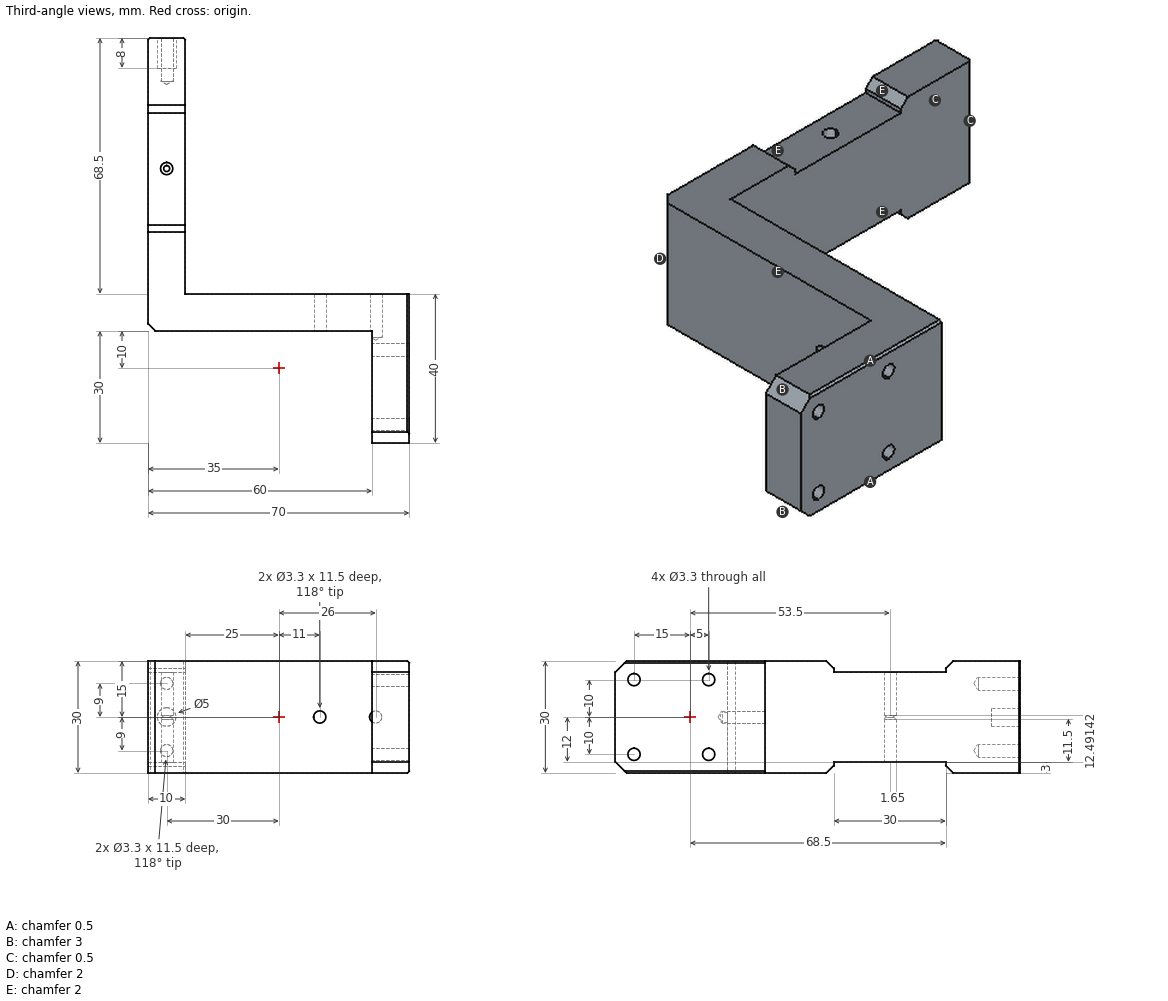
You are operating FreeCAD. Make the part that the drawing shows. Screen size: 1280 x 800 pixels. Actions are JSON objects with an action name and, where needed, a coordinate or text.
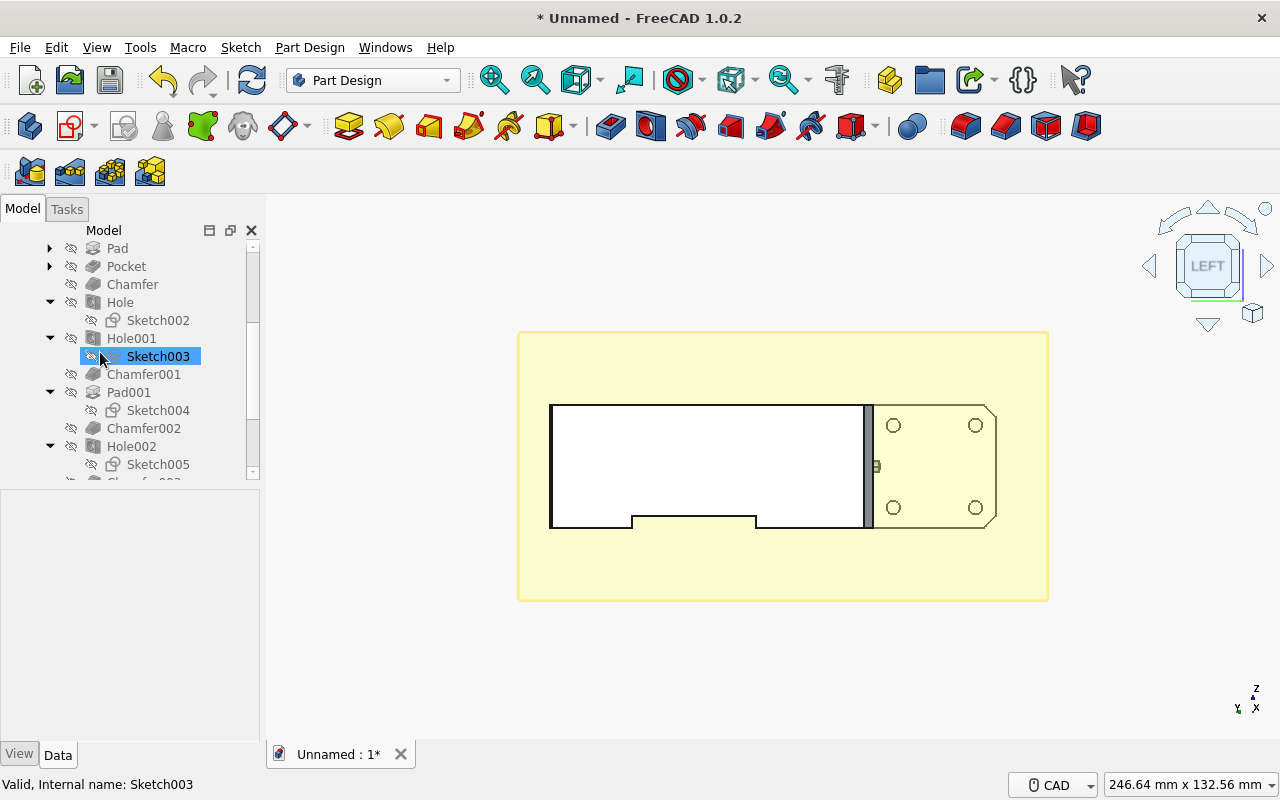
{"action": "scroll", "coordinate": [140, 352], "scroll_direction": "up", "scroll_amount": 15}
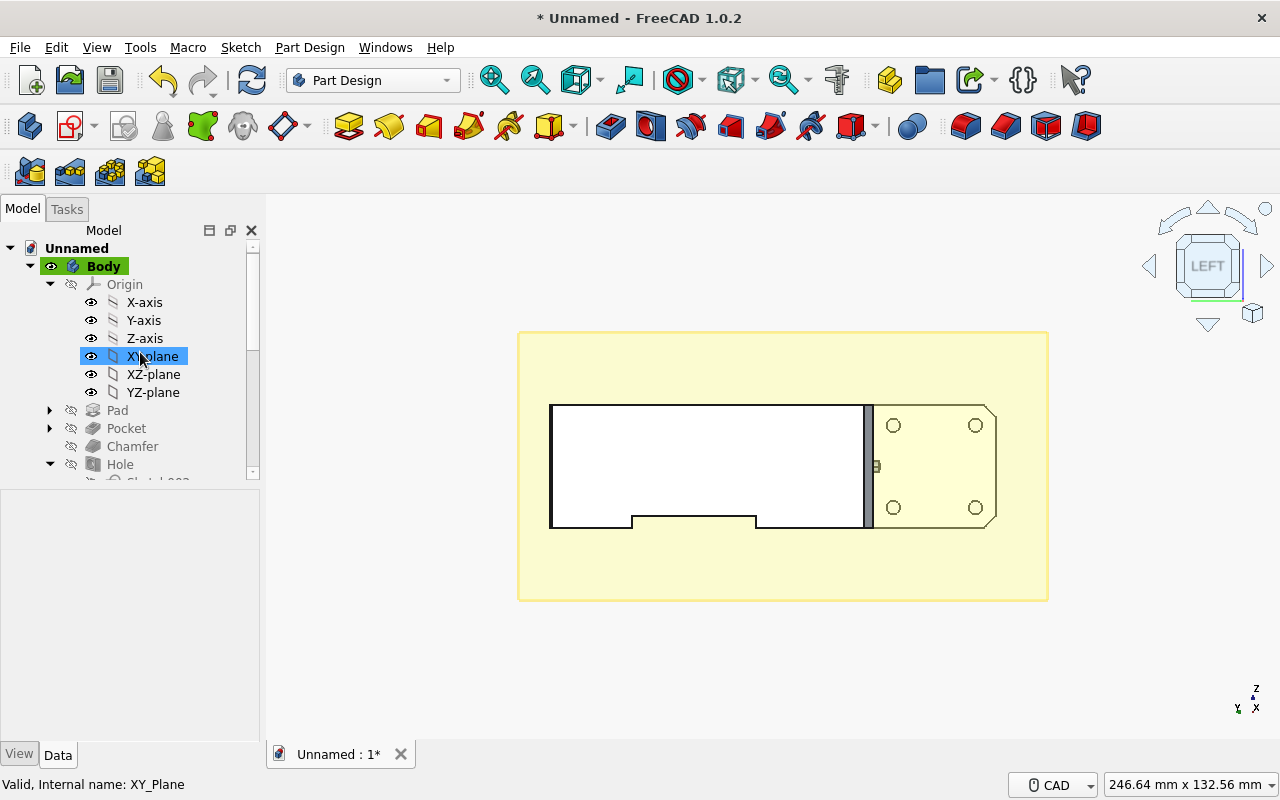
{"action": "scroll", "coordinate": [100, 352], "scroll_direction": "down", "scroll_amount": 6}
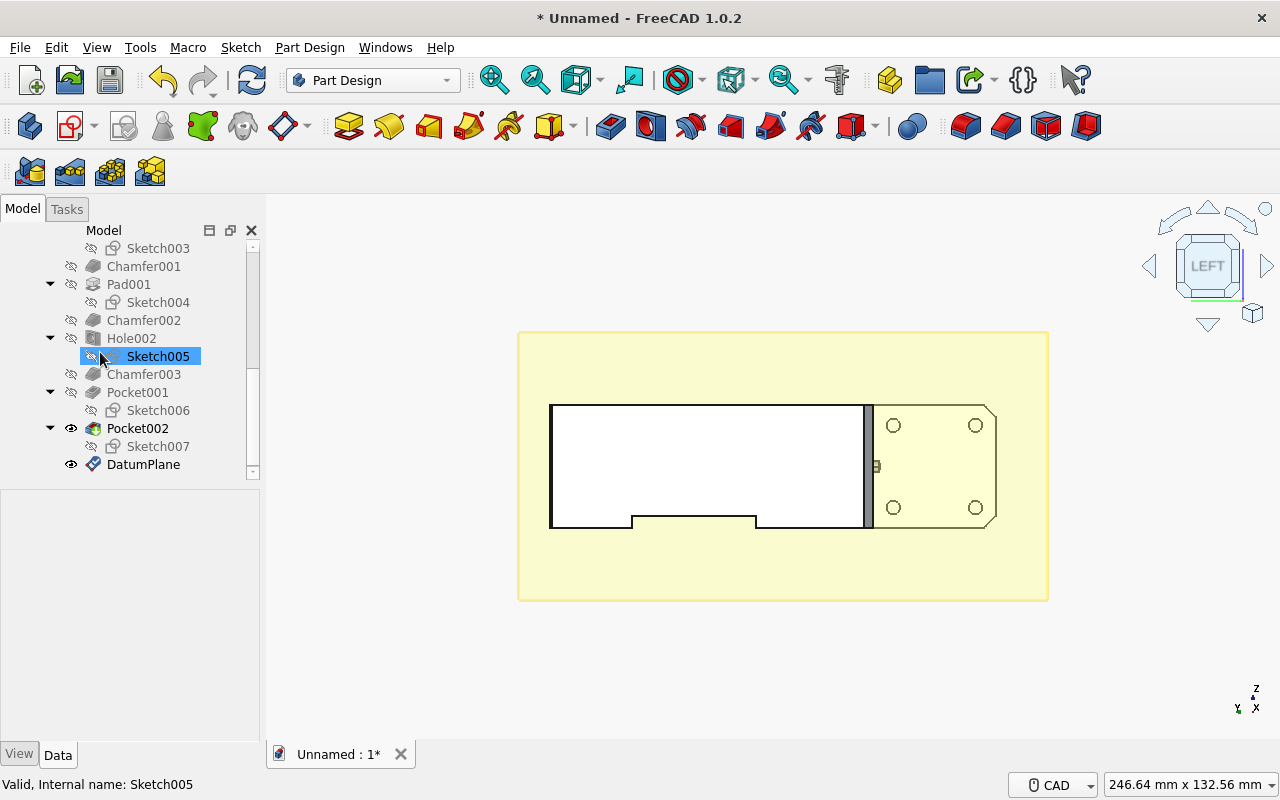
{"action": "left_click", "coordinate": [116, 464]}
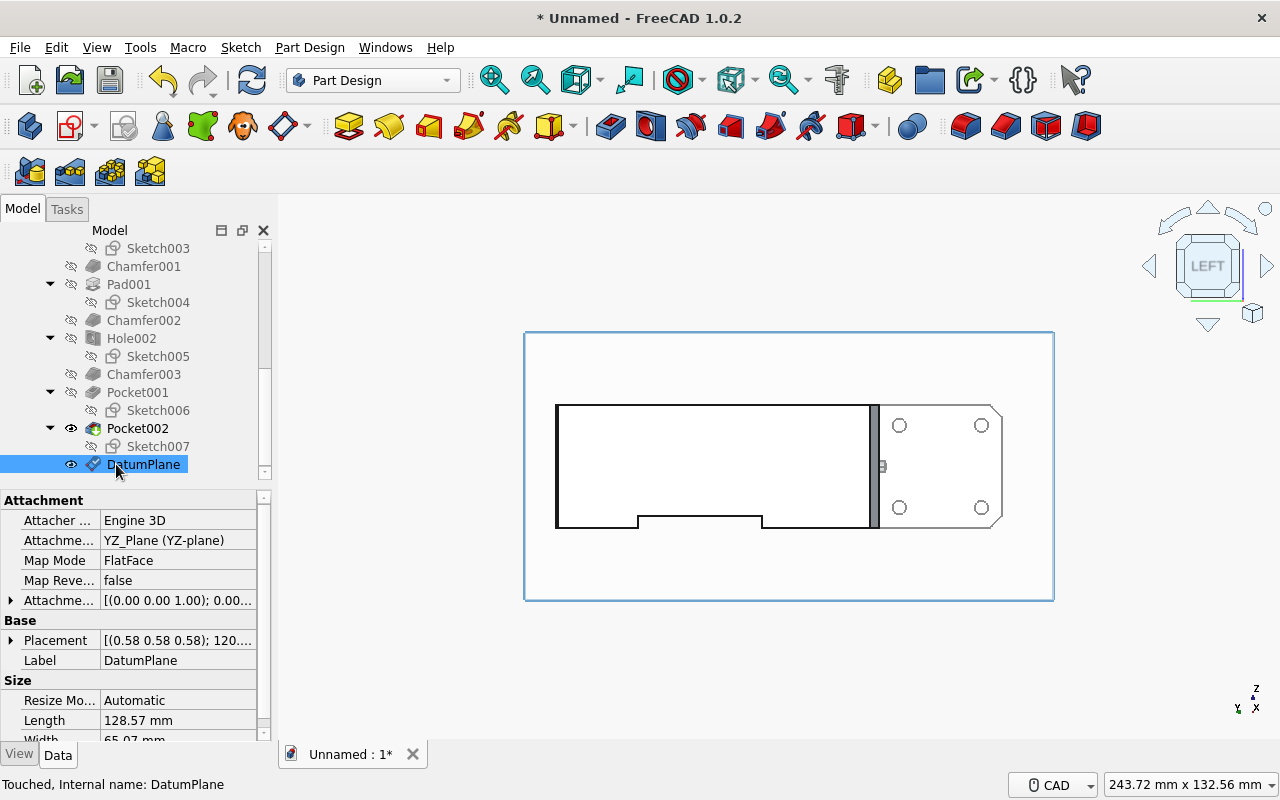
{"action": "left_click", "coordinate": [70, 126]}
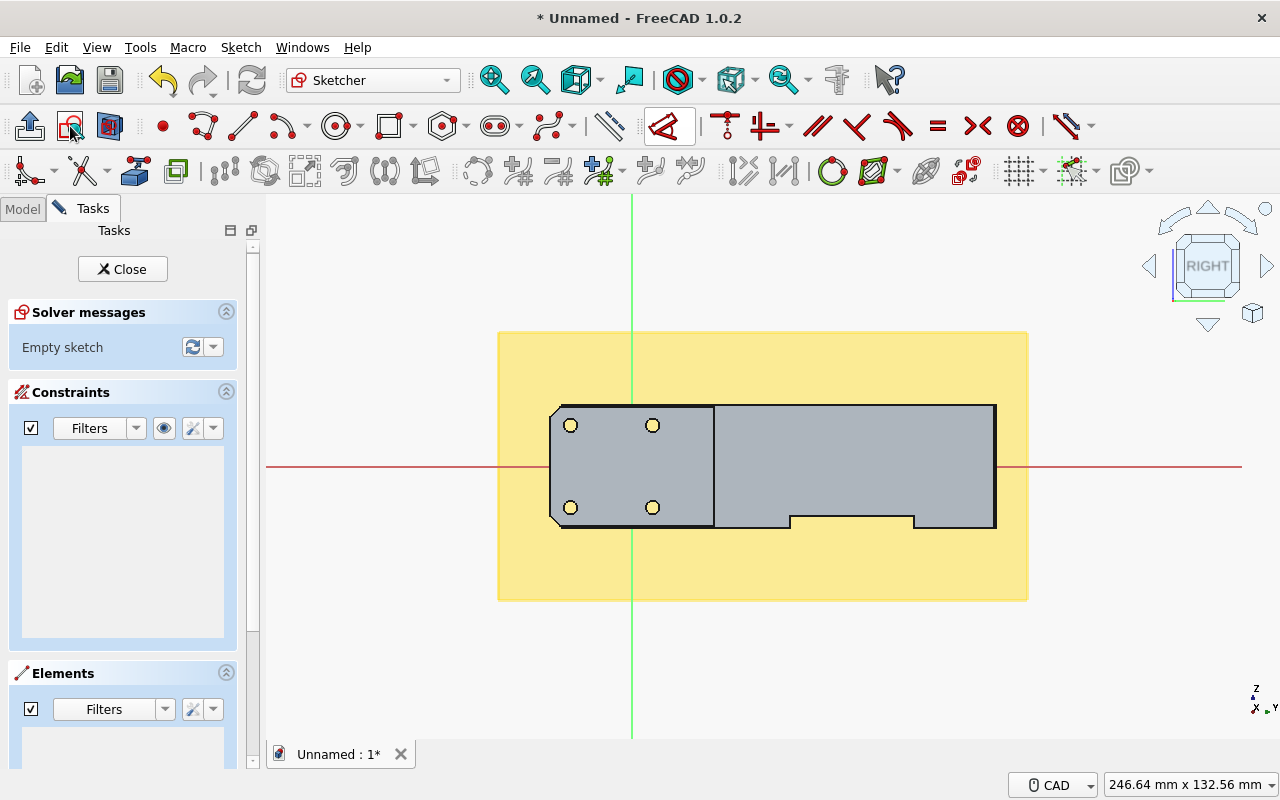
{"action": "left_click", "coordinate": [110, 126]}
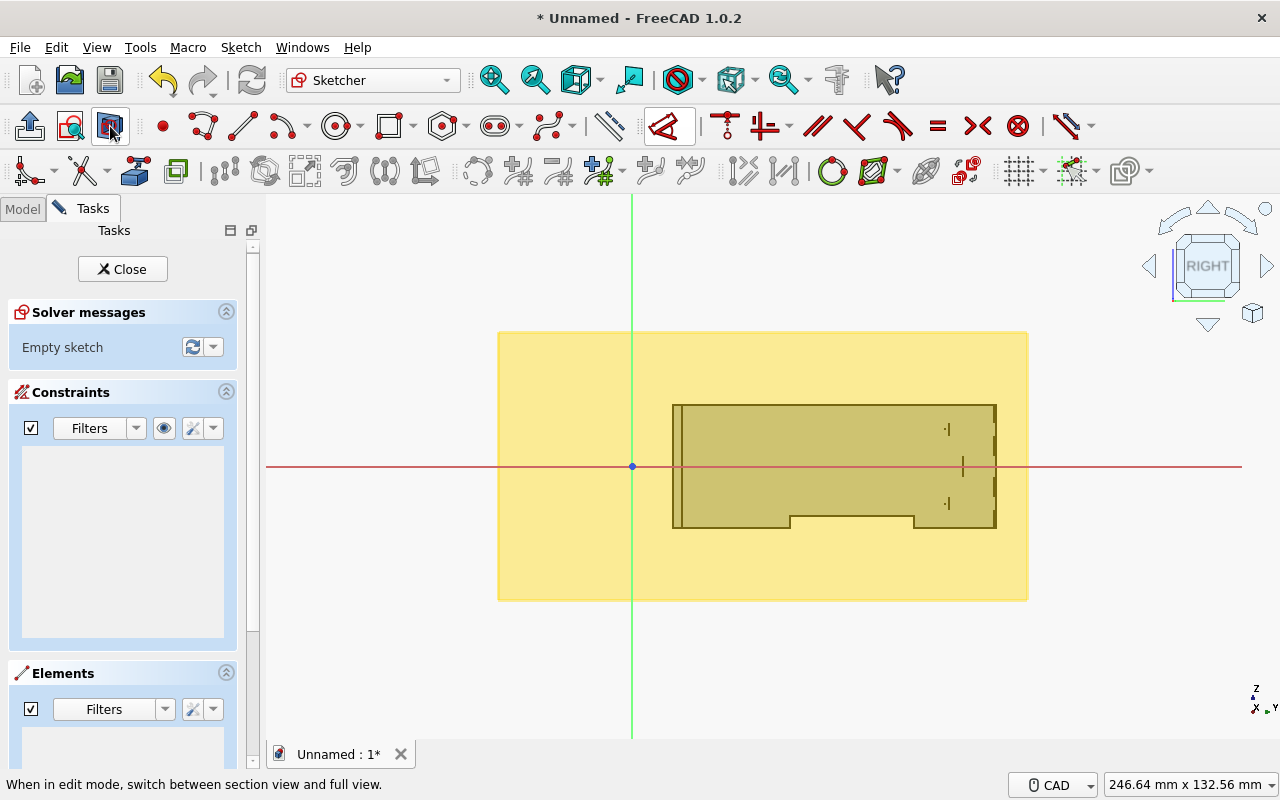
{"action": "scroll", "coordinate": [894, 483], "scroll_direction": "up", "scroll_amount": 8}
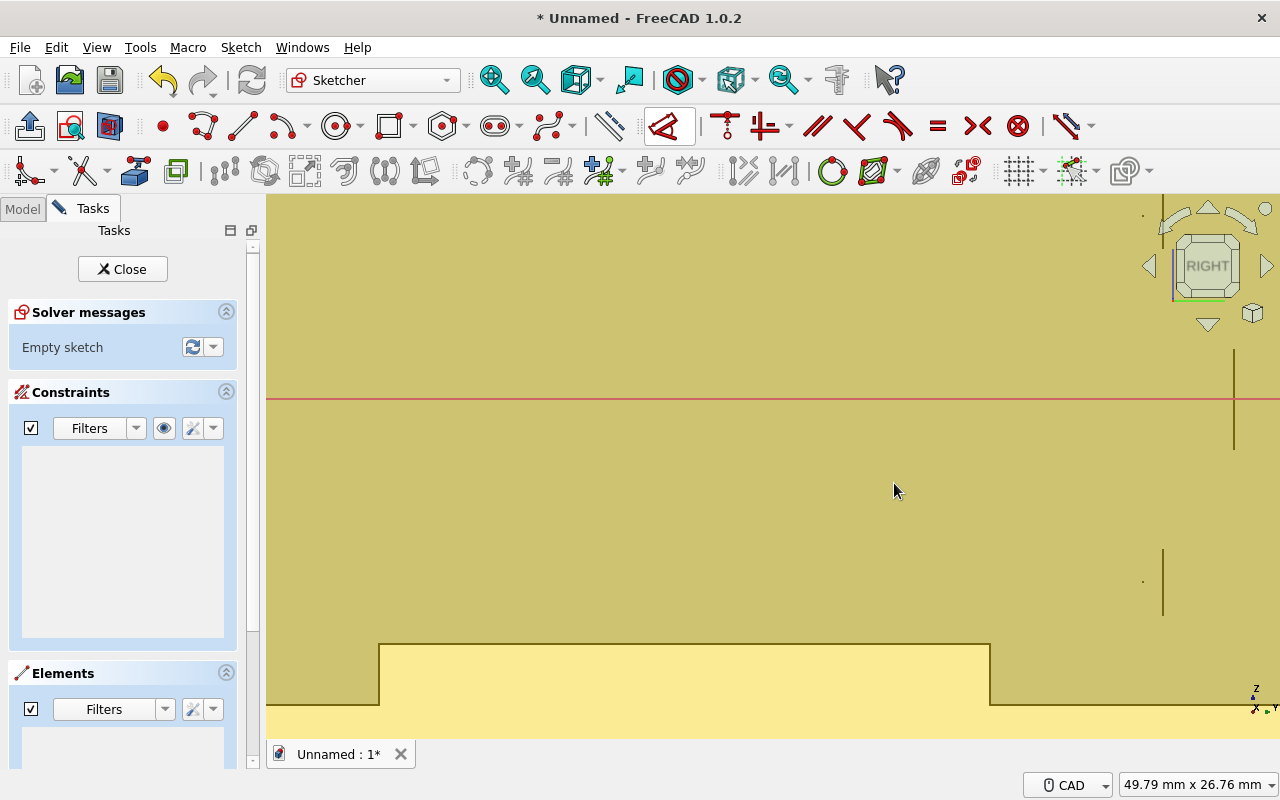
{"action": "key", "text": "g m"}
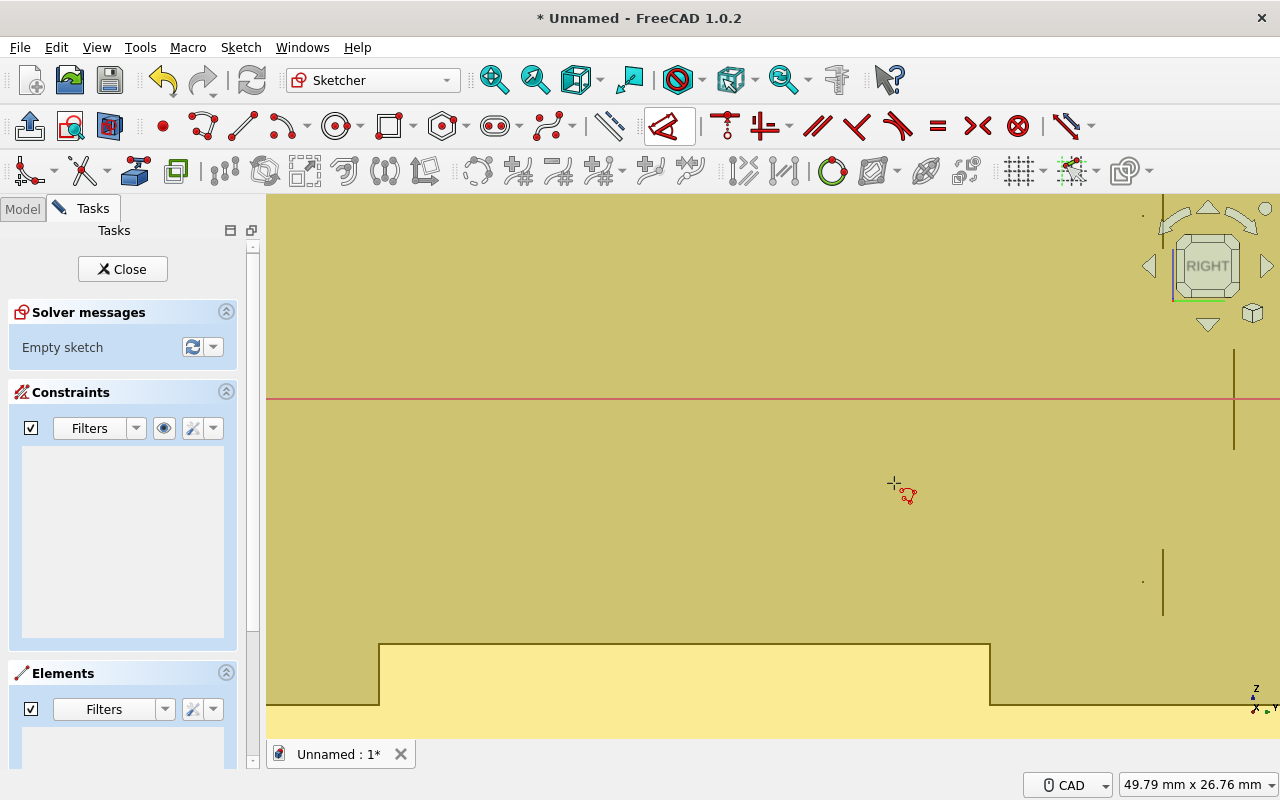
{"action": "scroll", "coordinate": [684, 389], "scroll_direction": "up", "scroll_amount": 3}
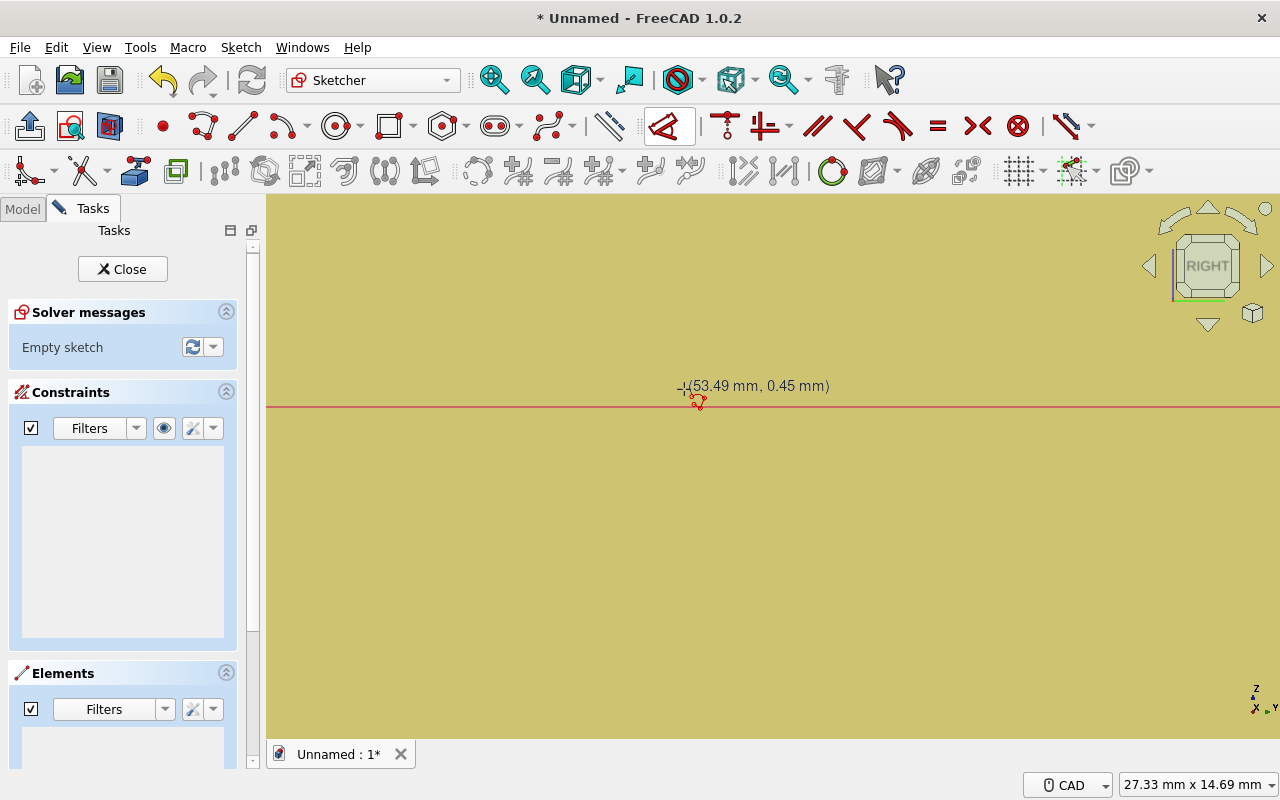
{"action": "left_click", "coordinate": [684, 389]}